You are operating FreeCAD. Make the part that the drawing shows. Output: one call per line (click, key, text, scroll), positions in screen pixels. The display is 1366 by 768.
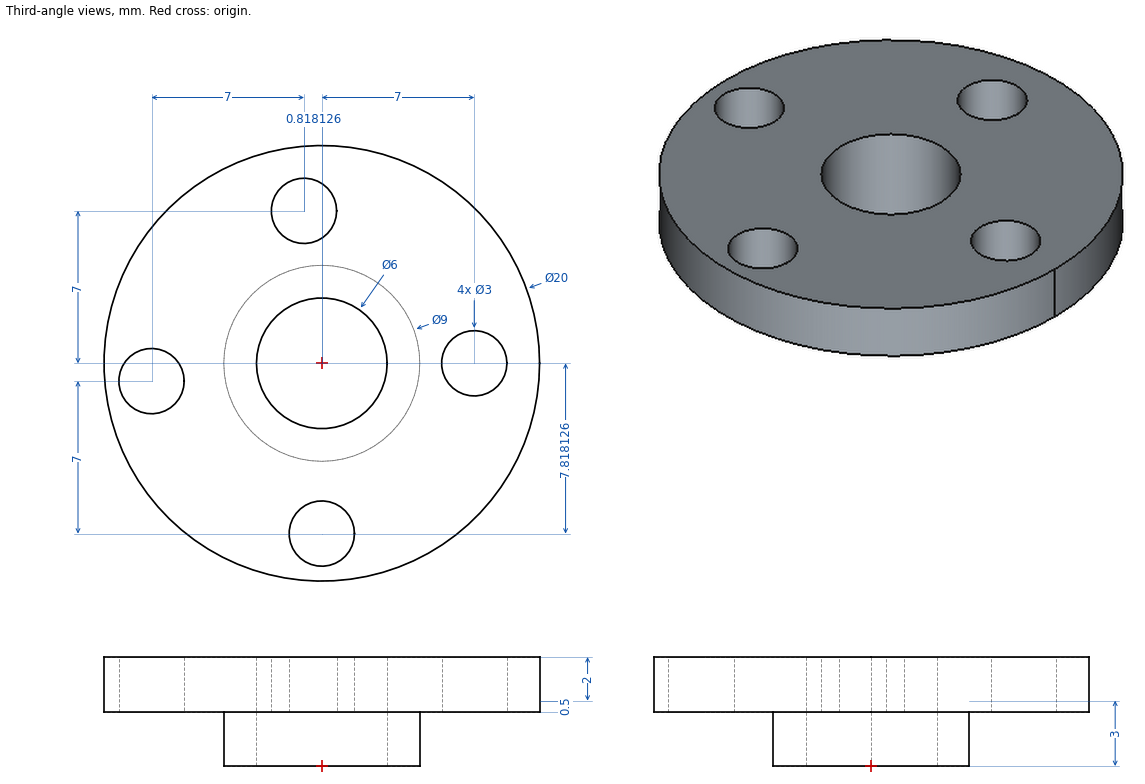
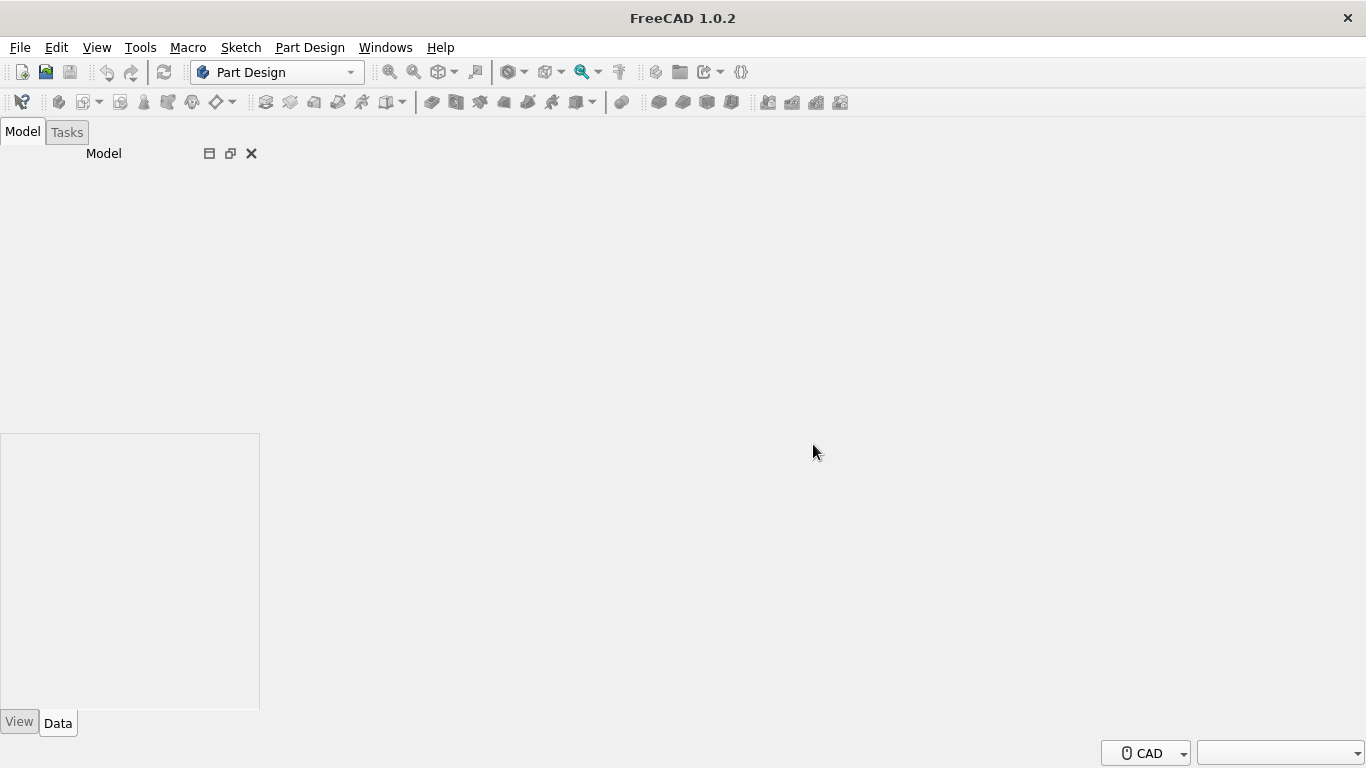
click(22, 72)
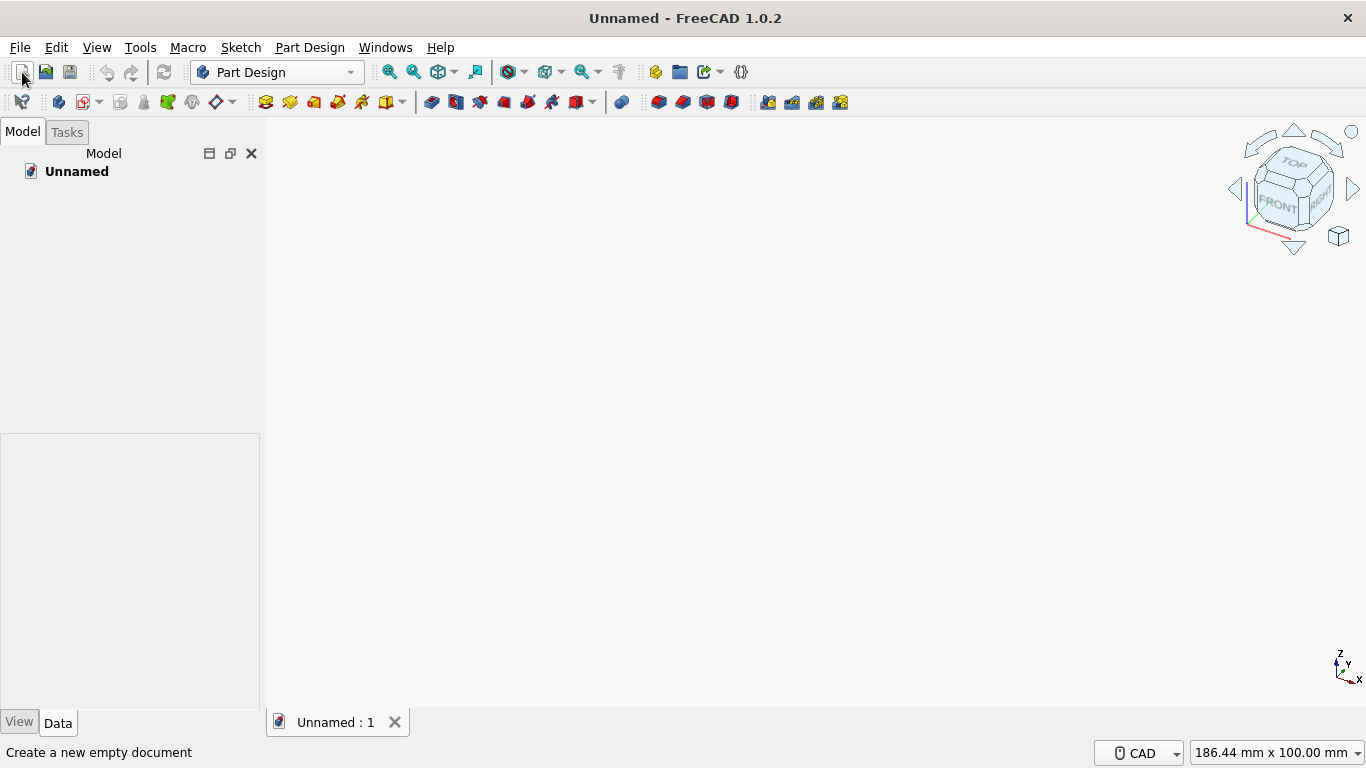
click(84, 102)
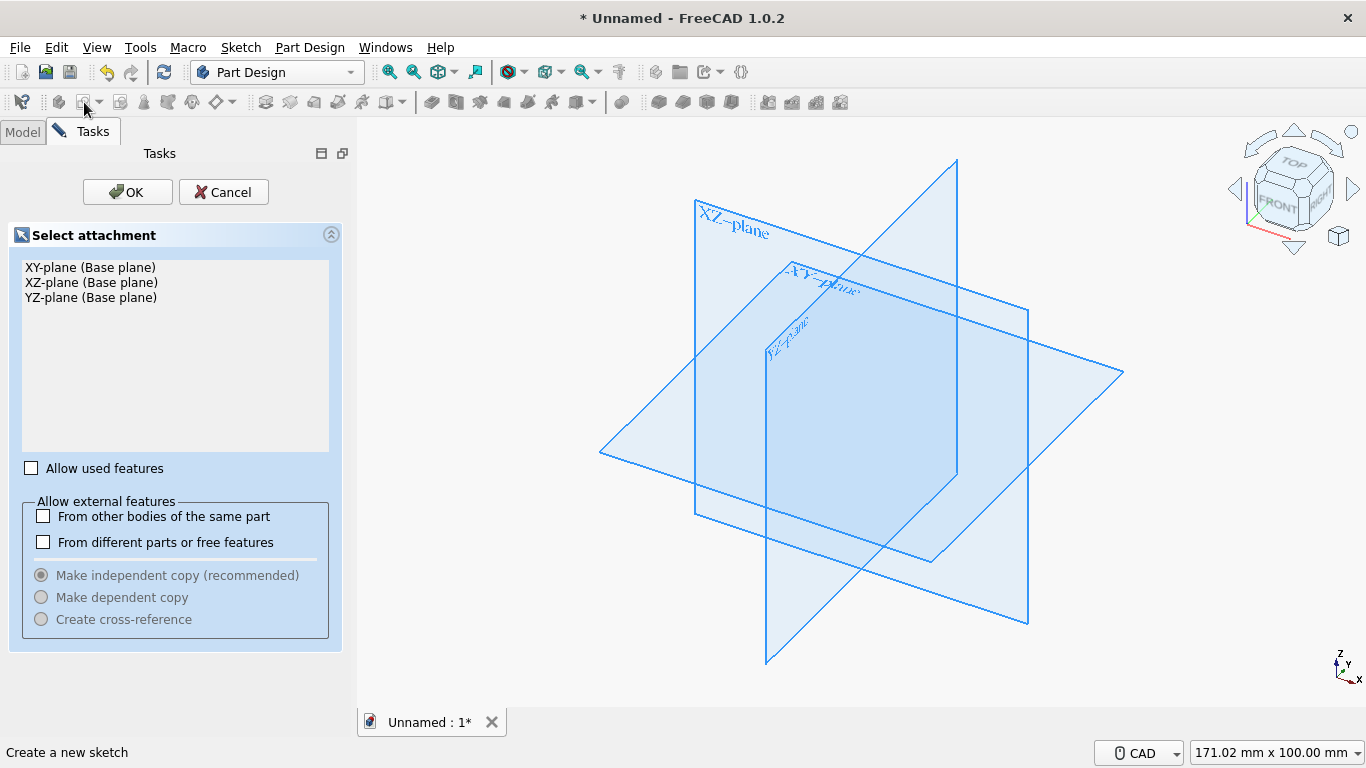
click(82, 268)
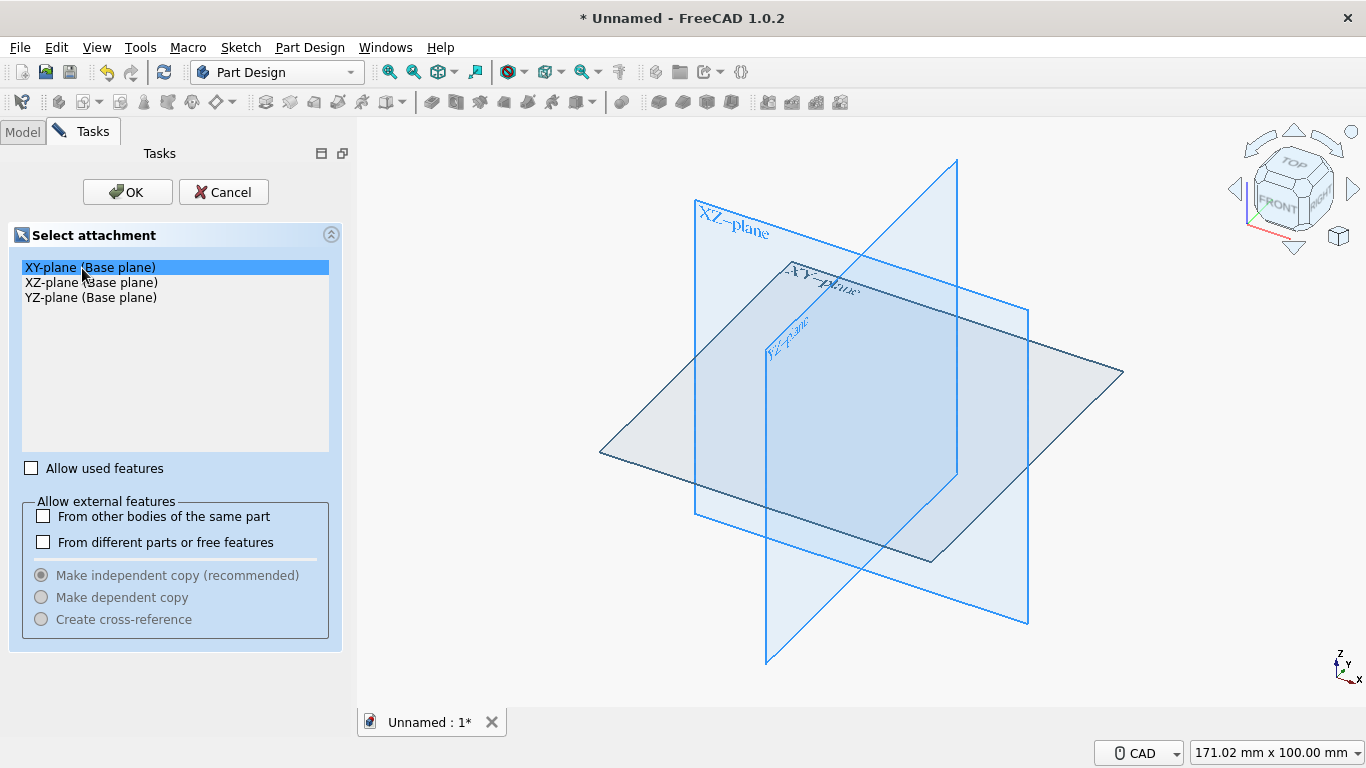
click(128, 192)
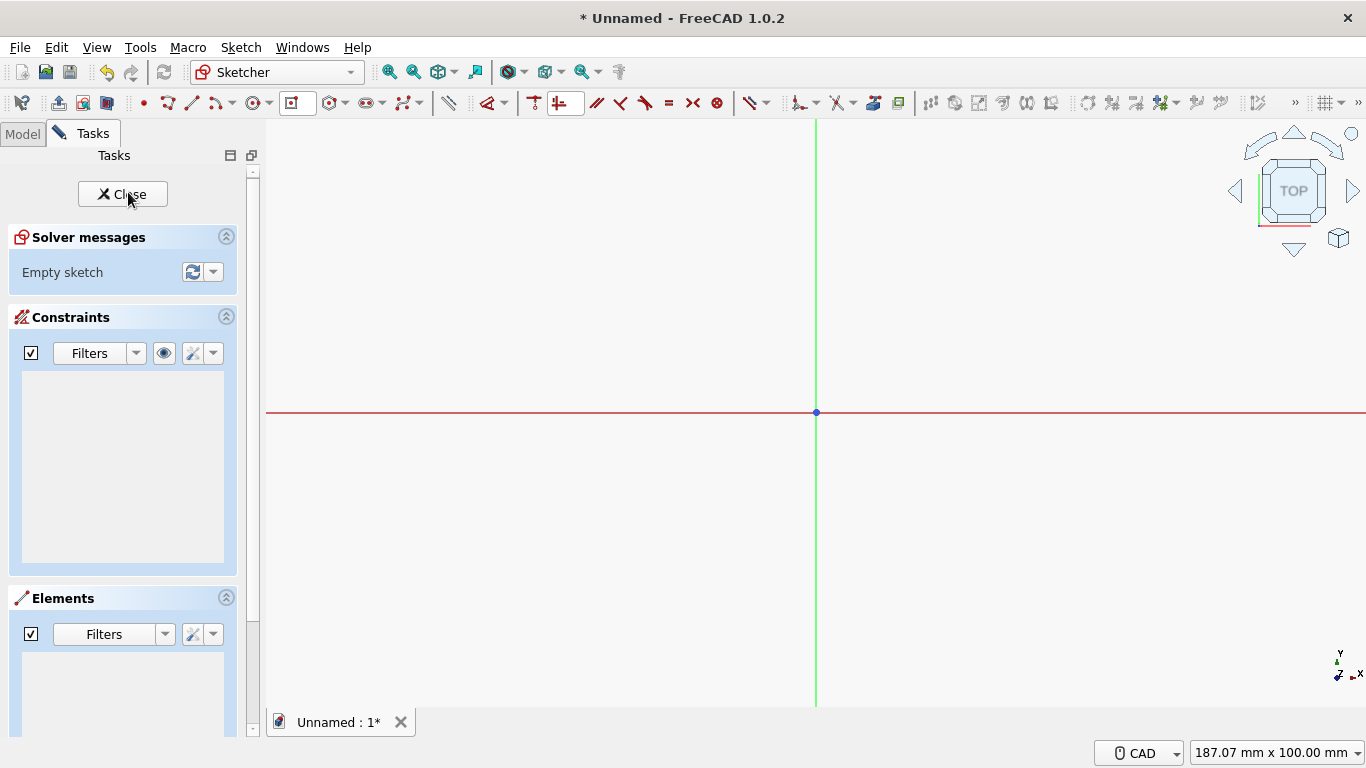
scroll(827, 413, up, 10)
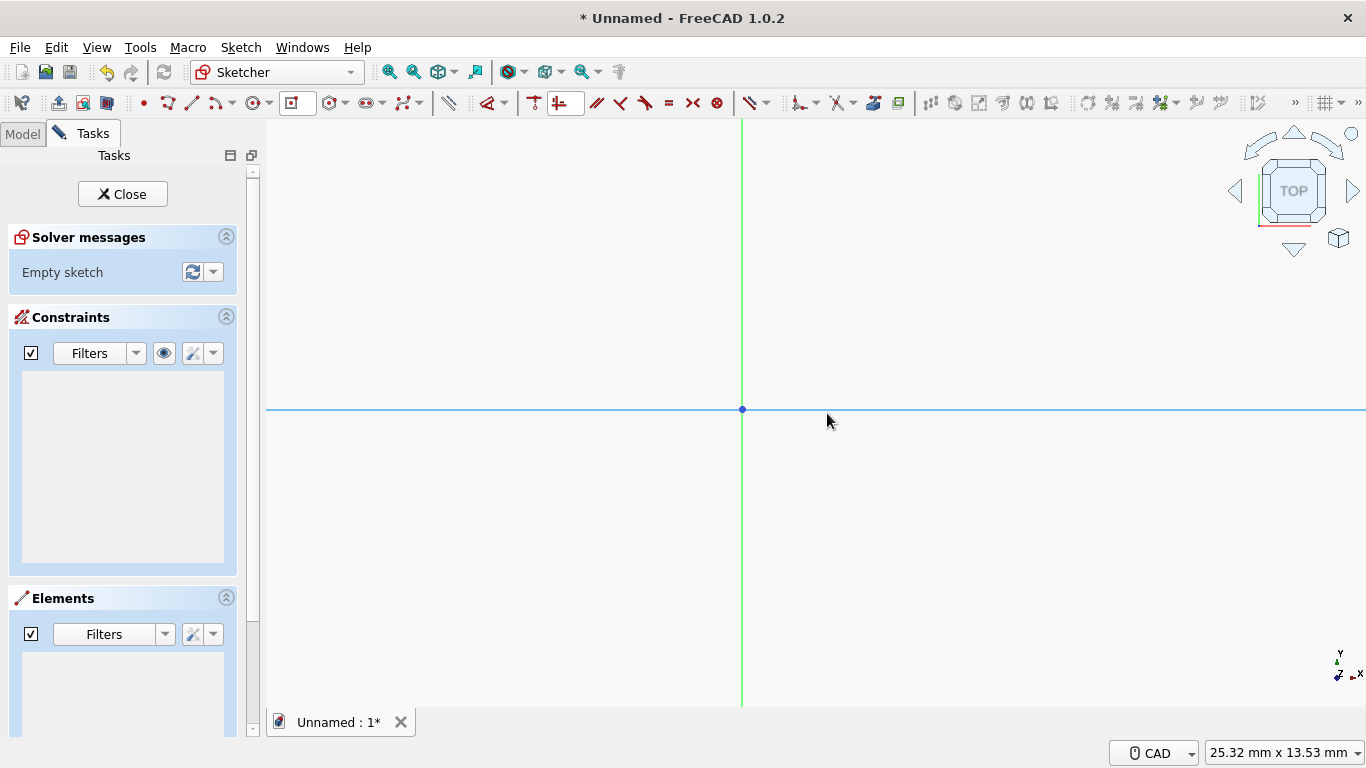
key(g)
key(c)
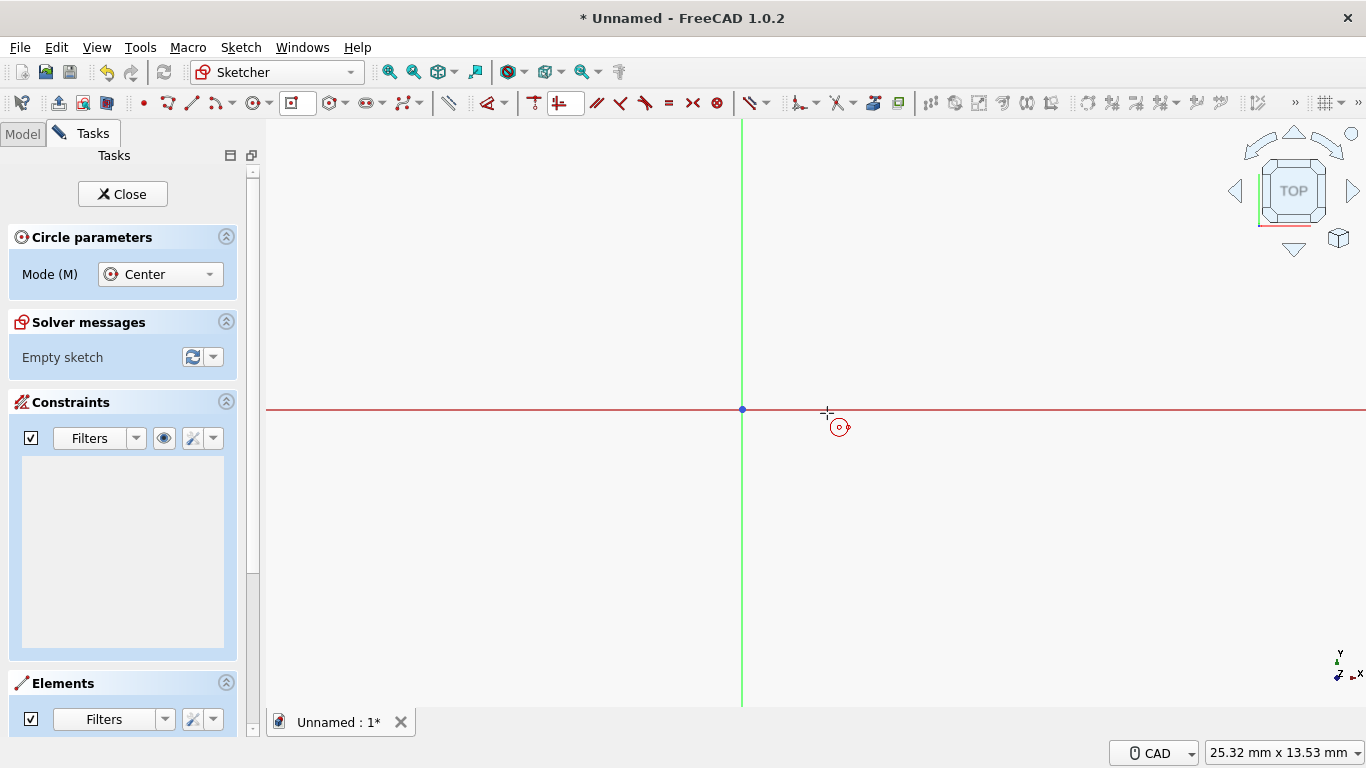
click(742, 410)
move(881, 272)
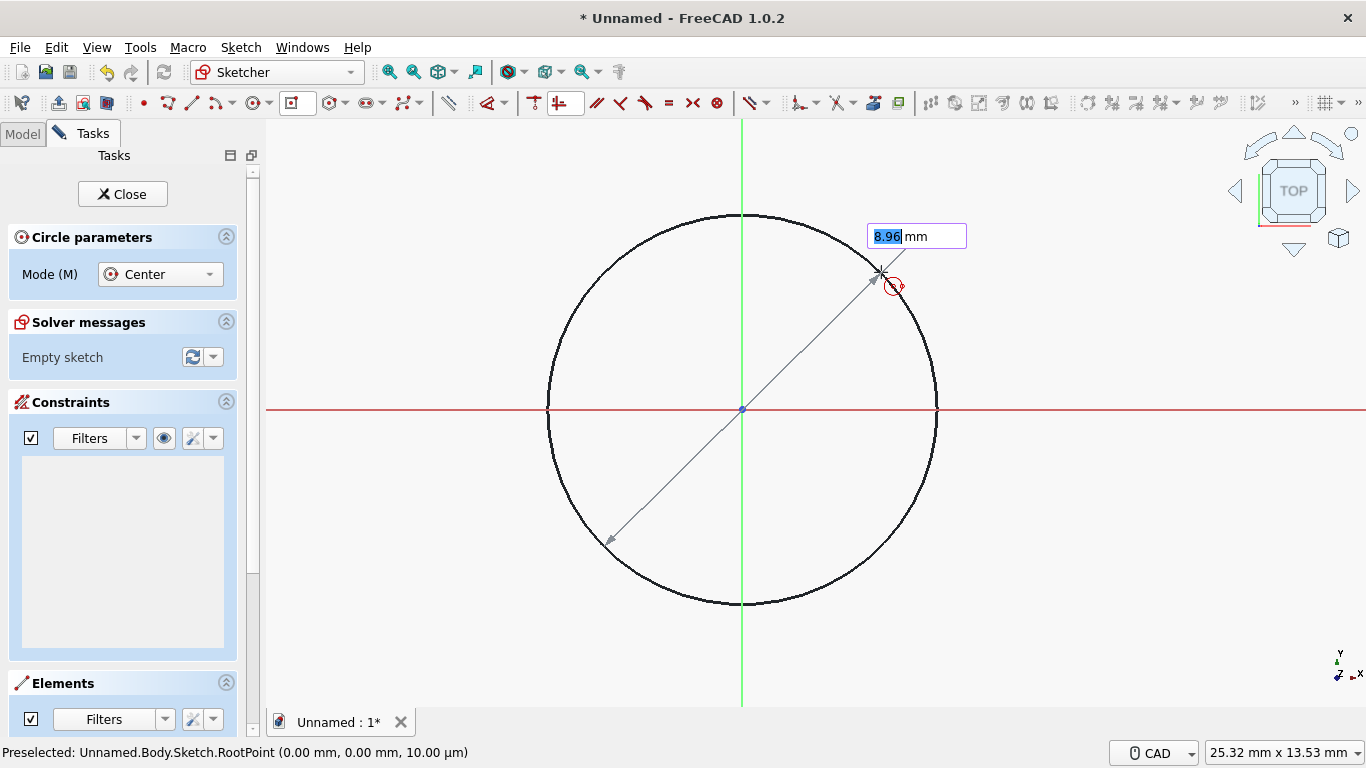
text(9)
key(Return)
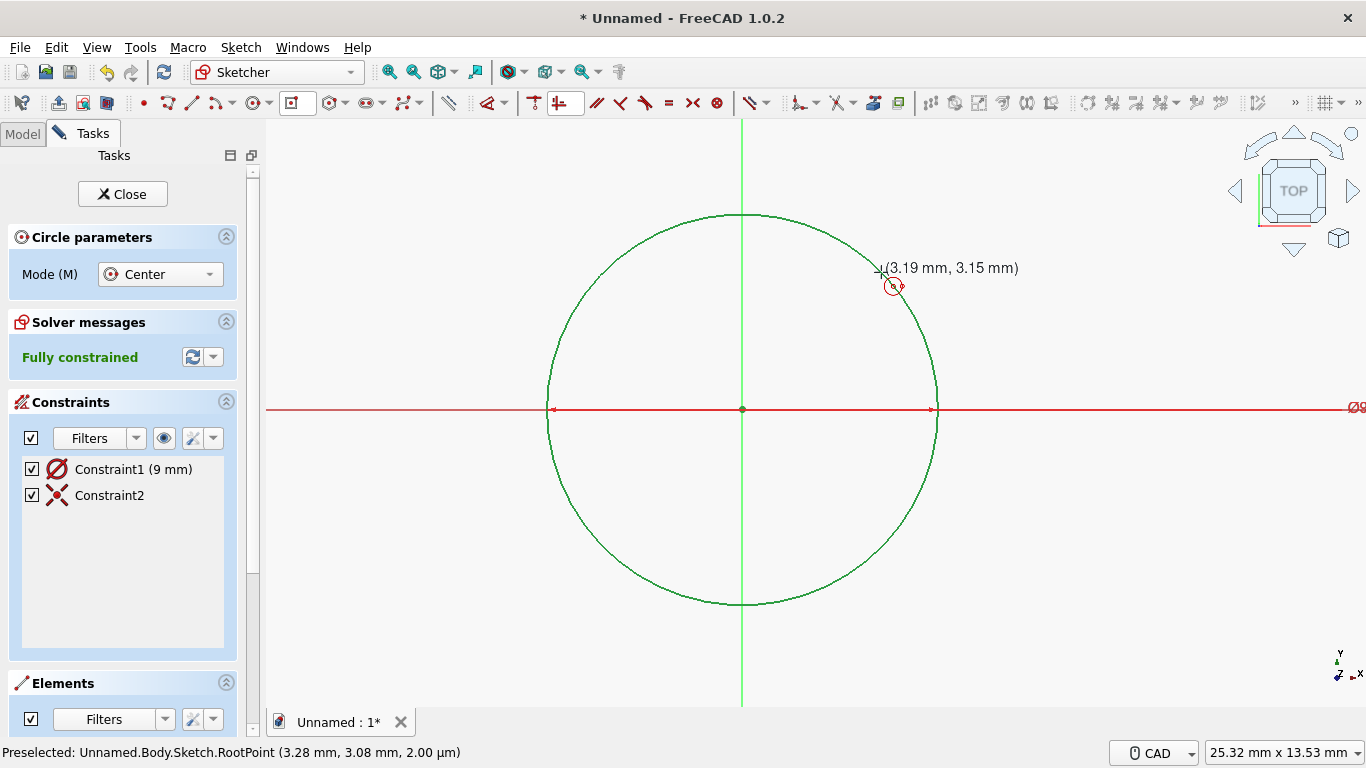
click(742, 410)
move(835, 318)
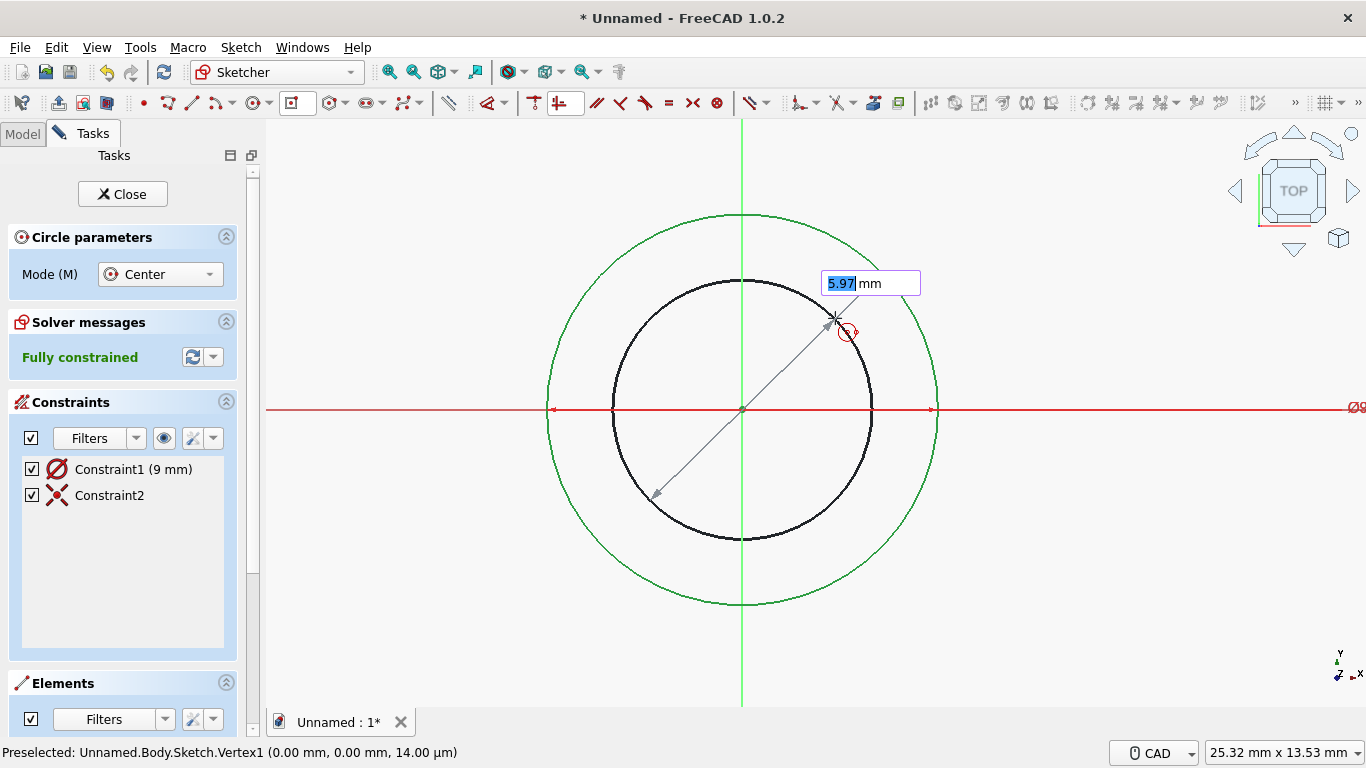
text(6)
key(Return)
key(Escape)